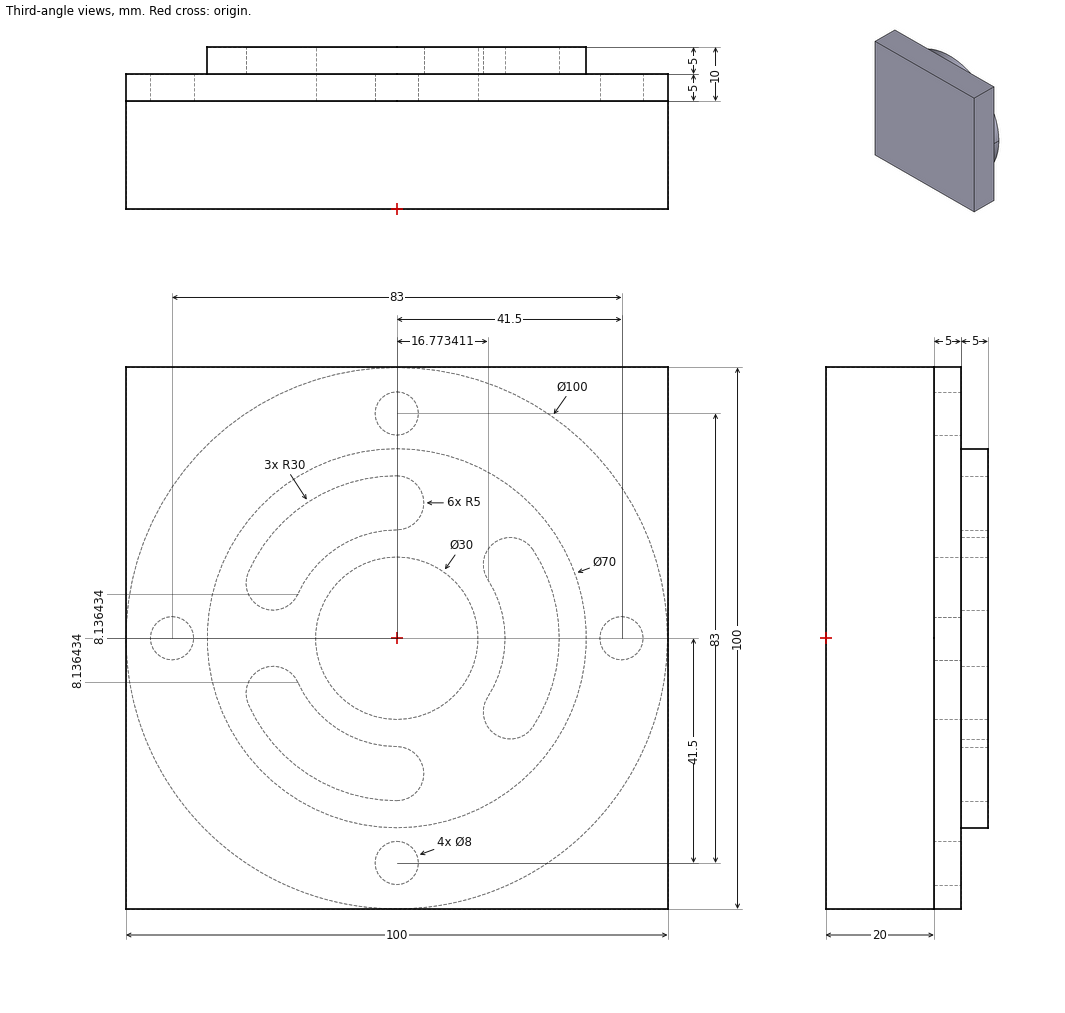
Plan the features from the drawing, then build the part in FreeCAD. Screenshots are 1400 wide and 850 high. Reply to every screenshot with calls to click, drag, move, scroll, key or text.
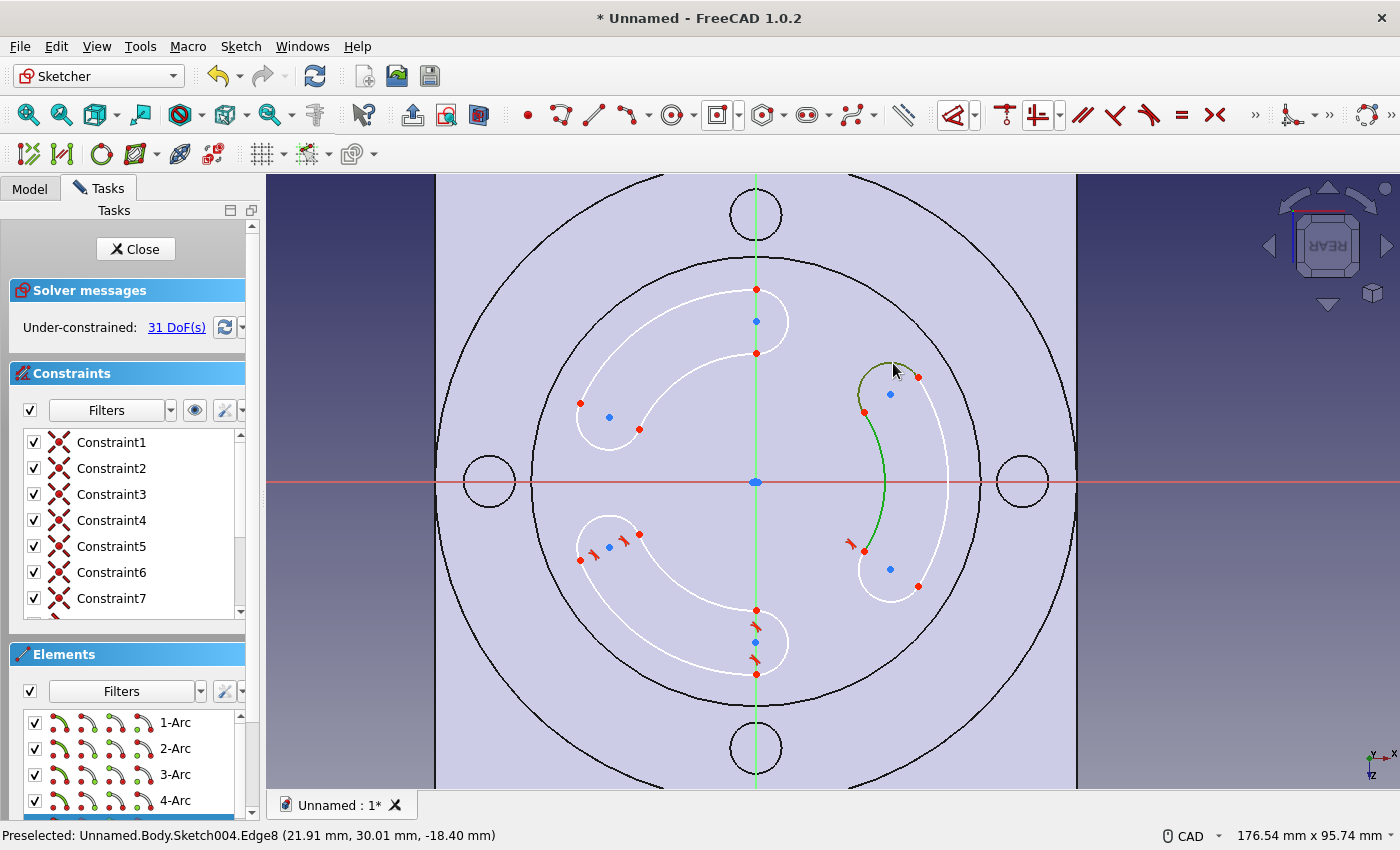
click(1149, 116)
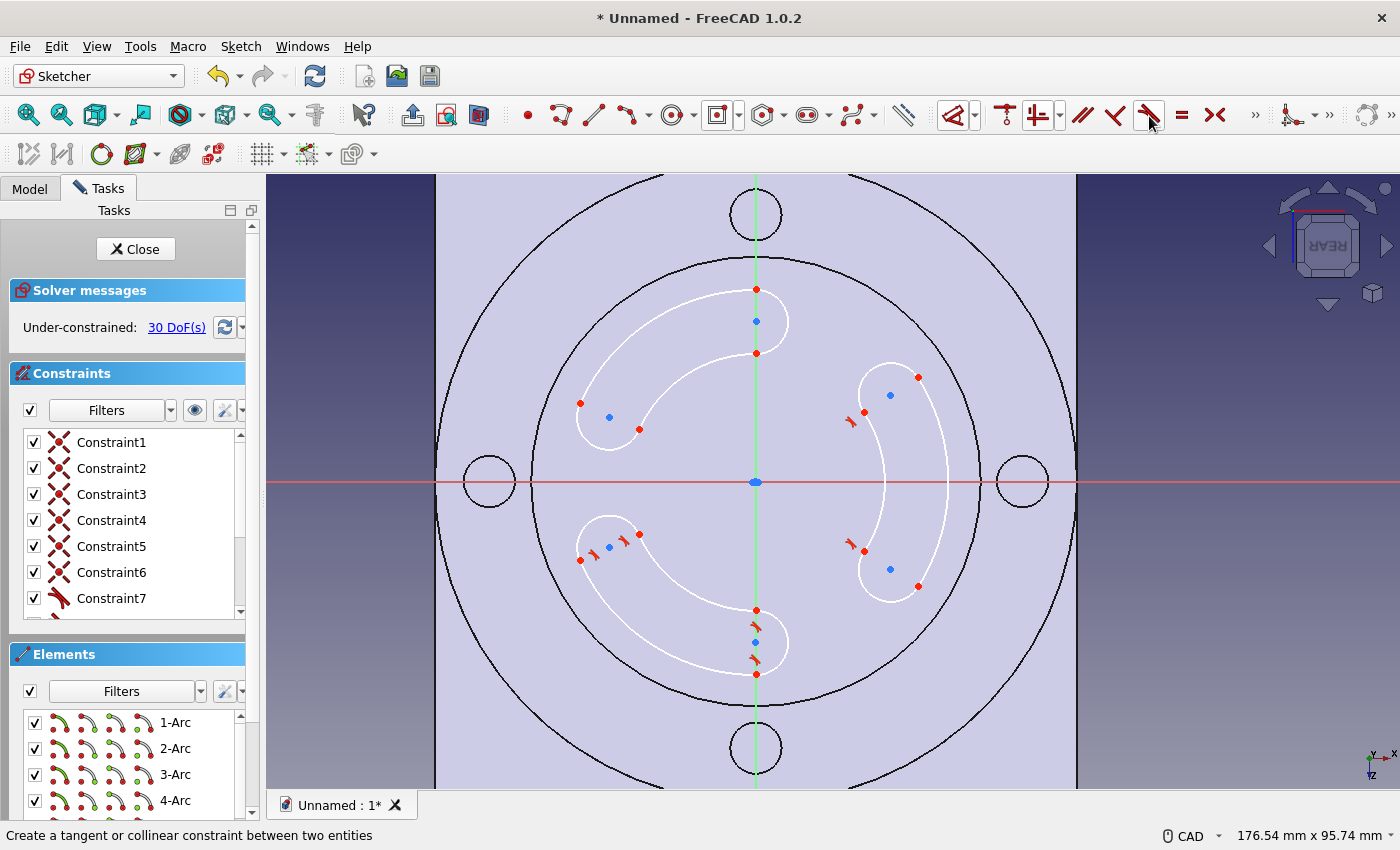
click(861, 581)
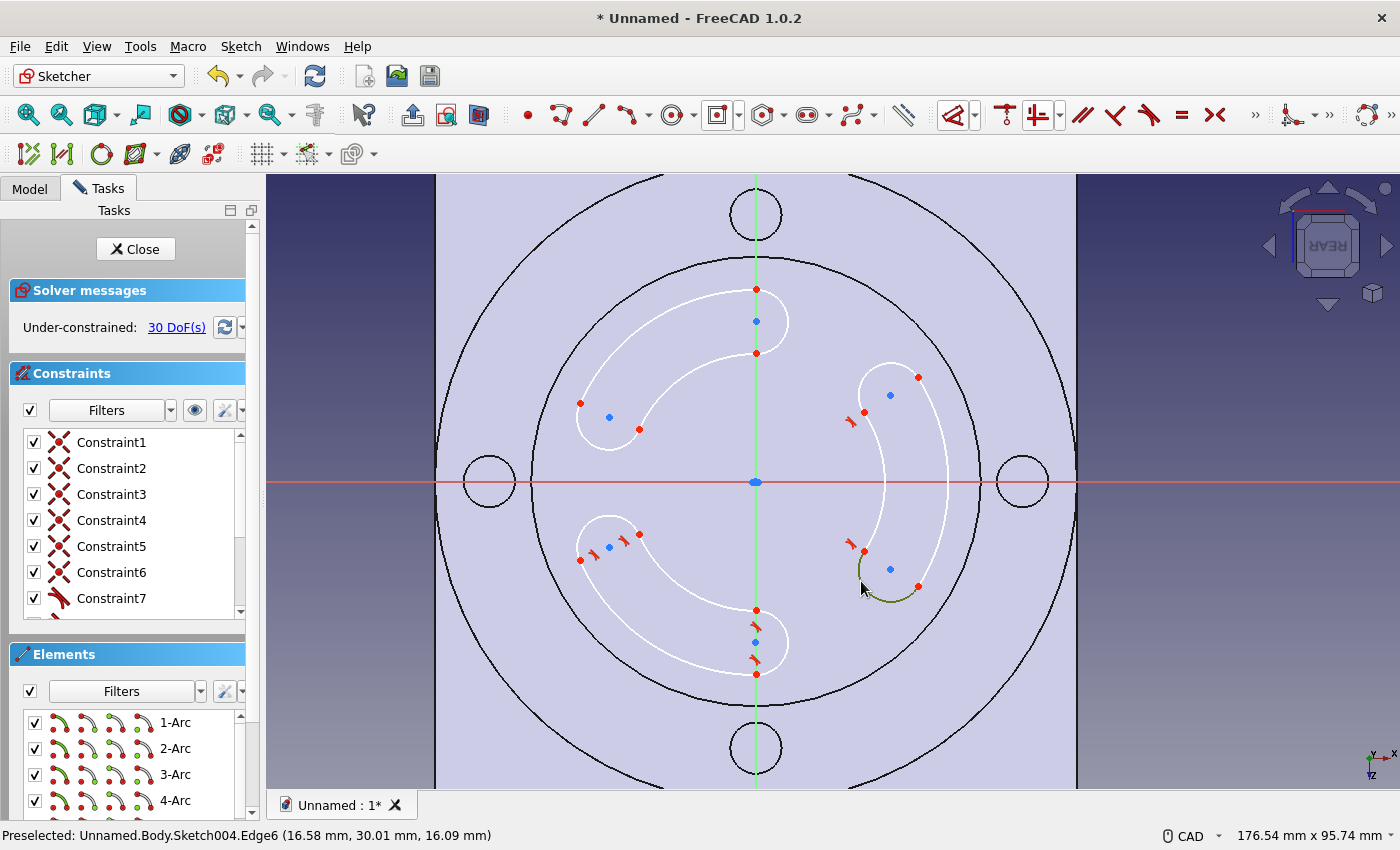
click(943, 526)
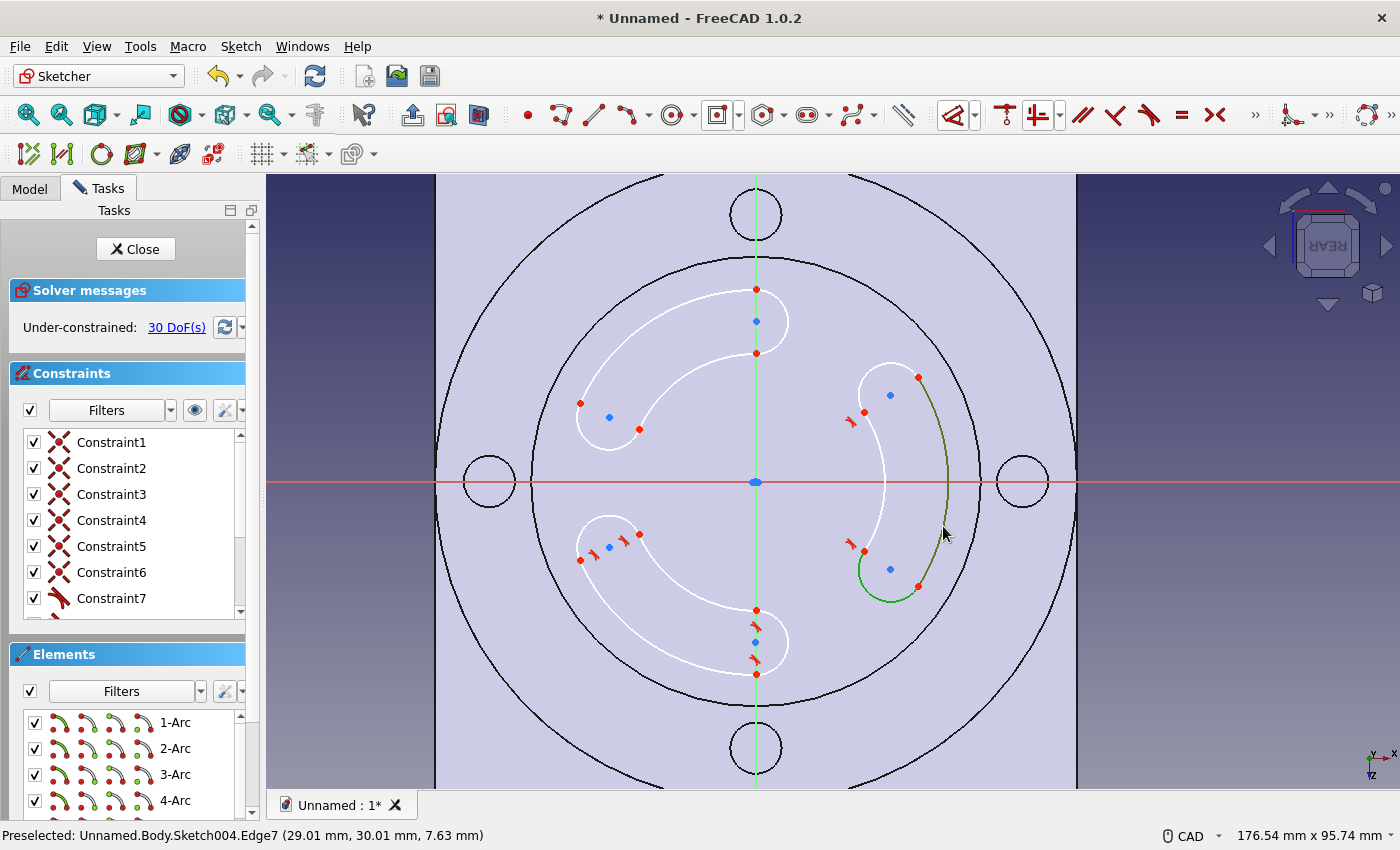
click(1149, 116)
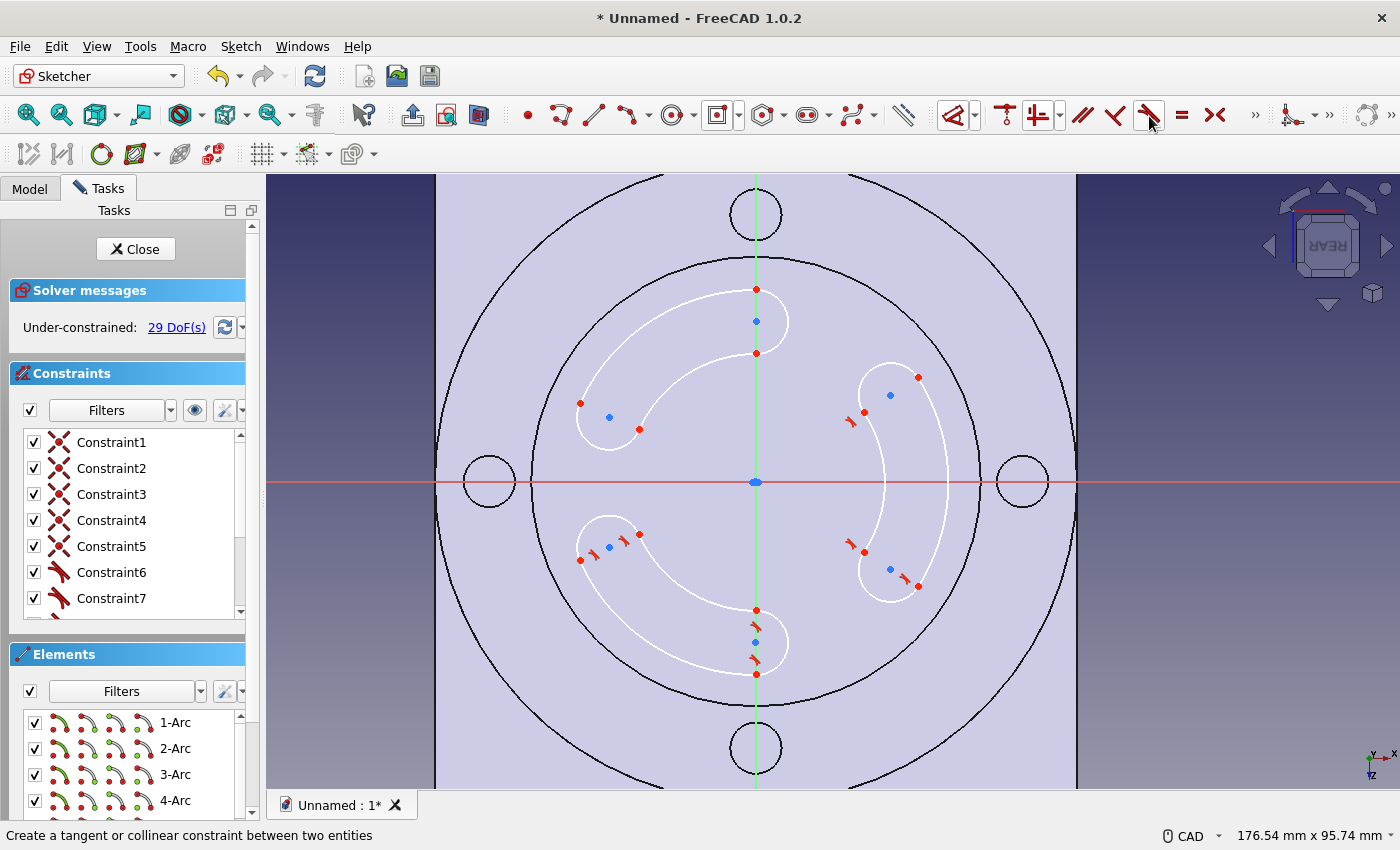
click(943, 526)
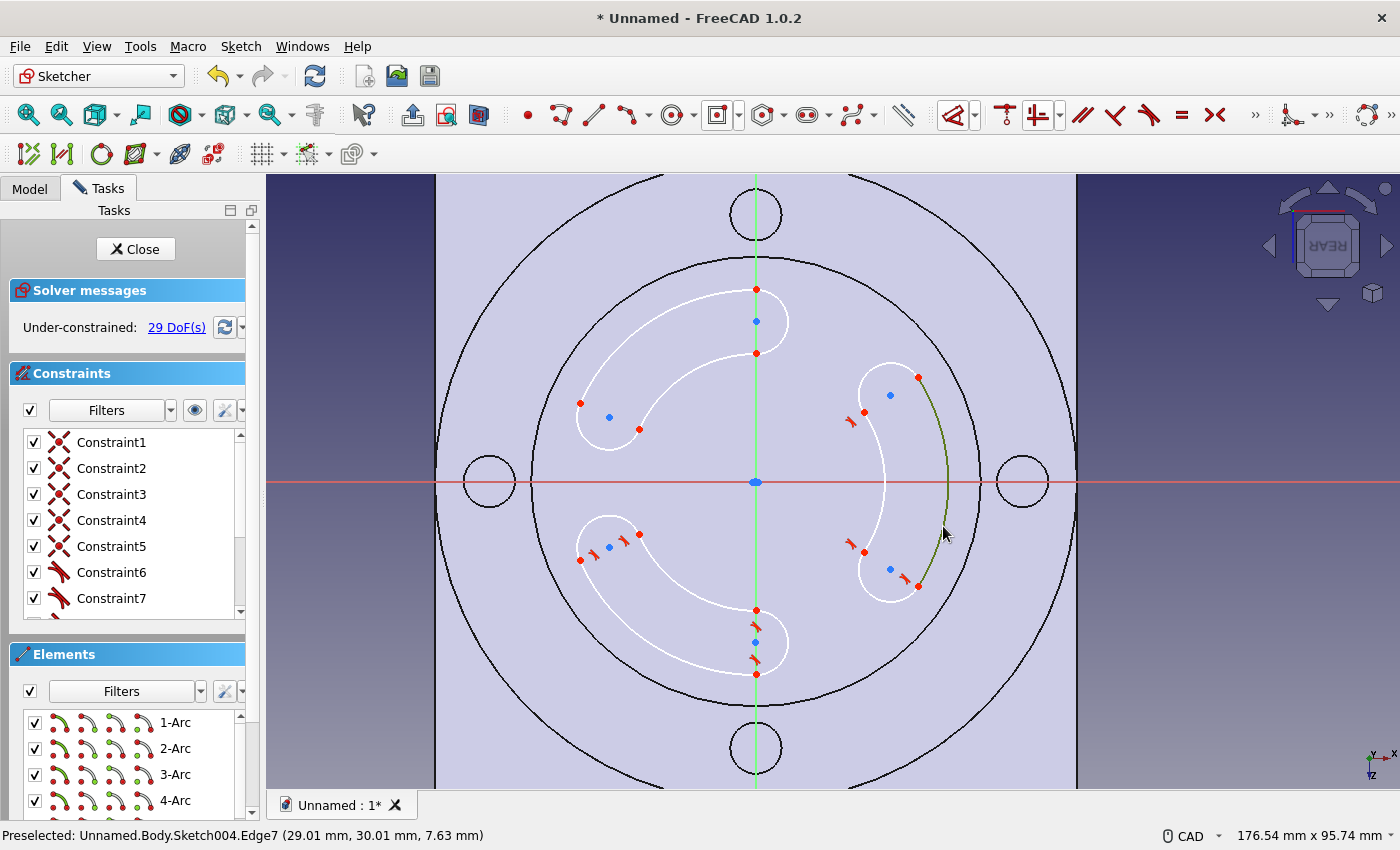
click(893, 363)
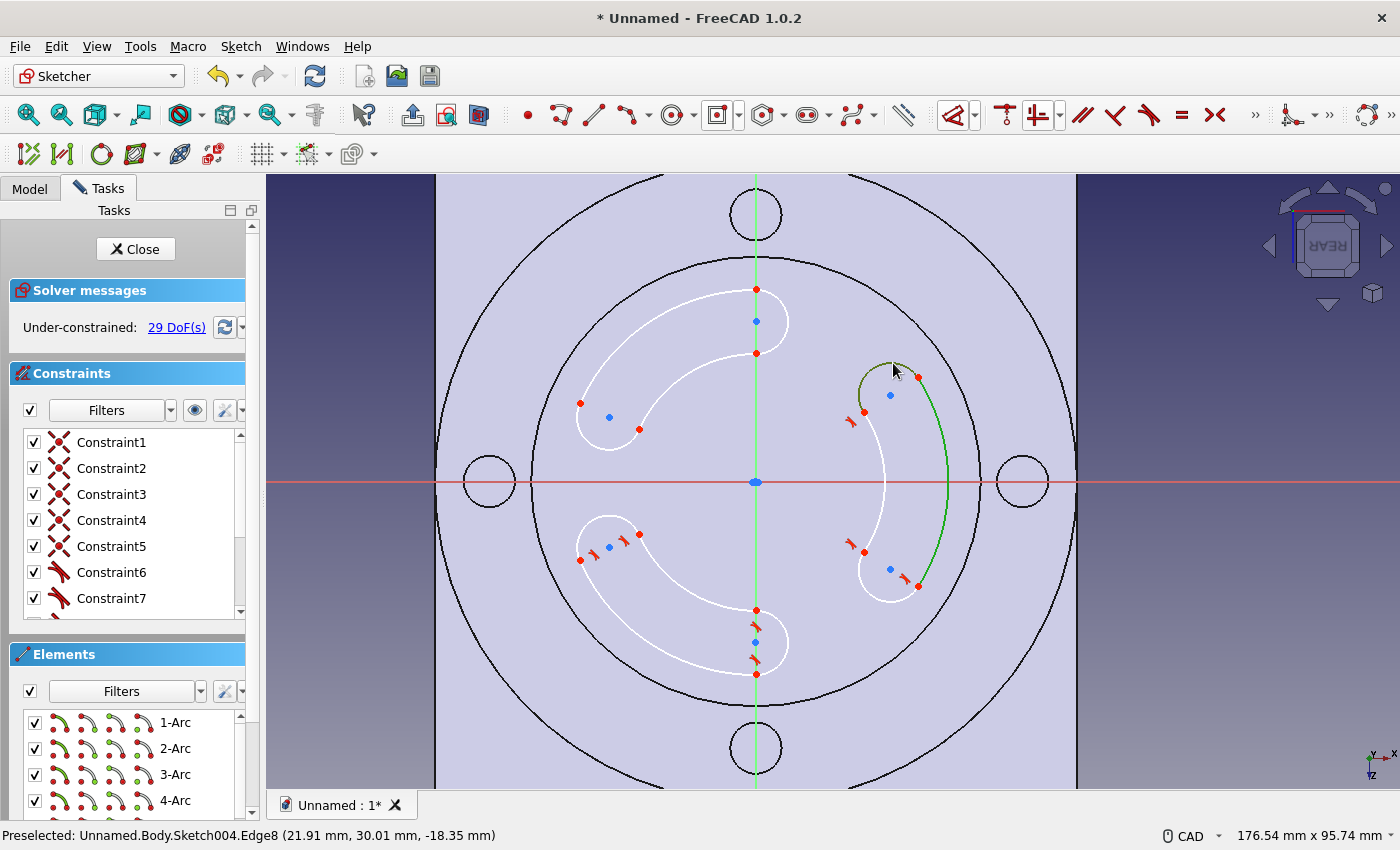
click(1149, 116)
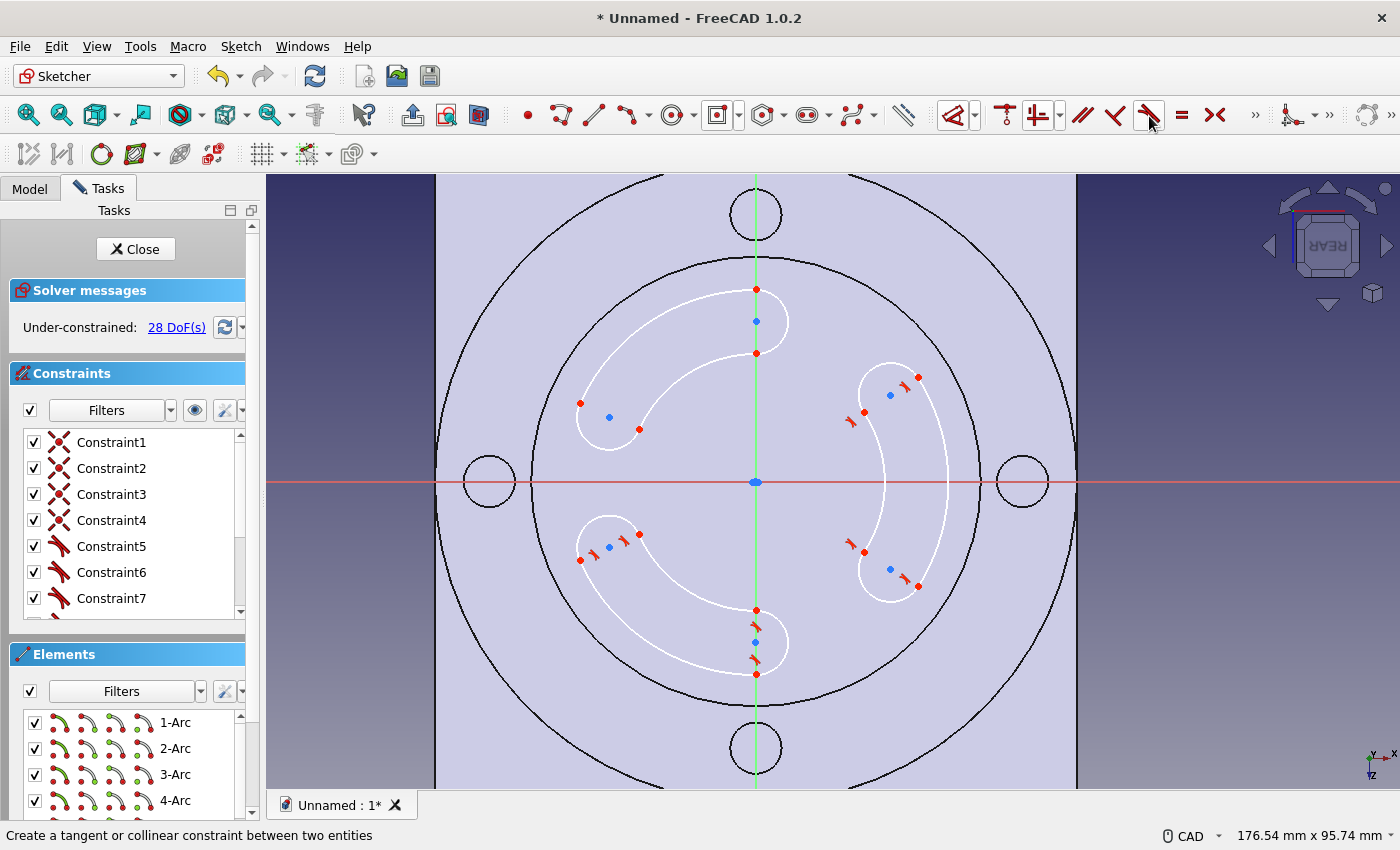
click(713, 362)